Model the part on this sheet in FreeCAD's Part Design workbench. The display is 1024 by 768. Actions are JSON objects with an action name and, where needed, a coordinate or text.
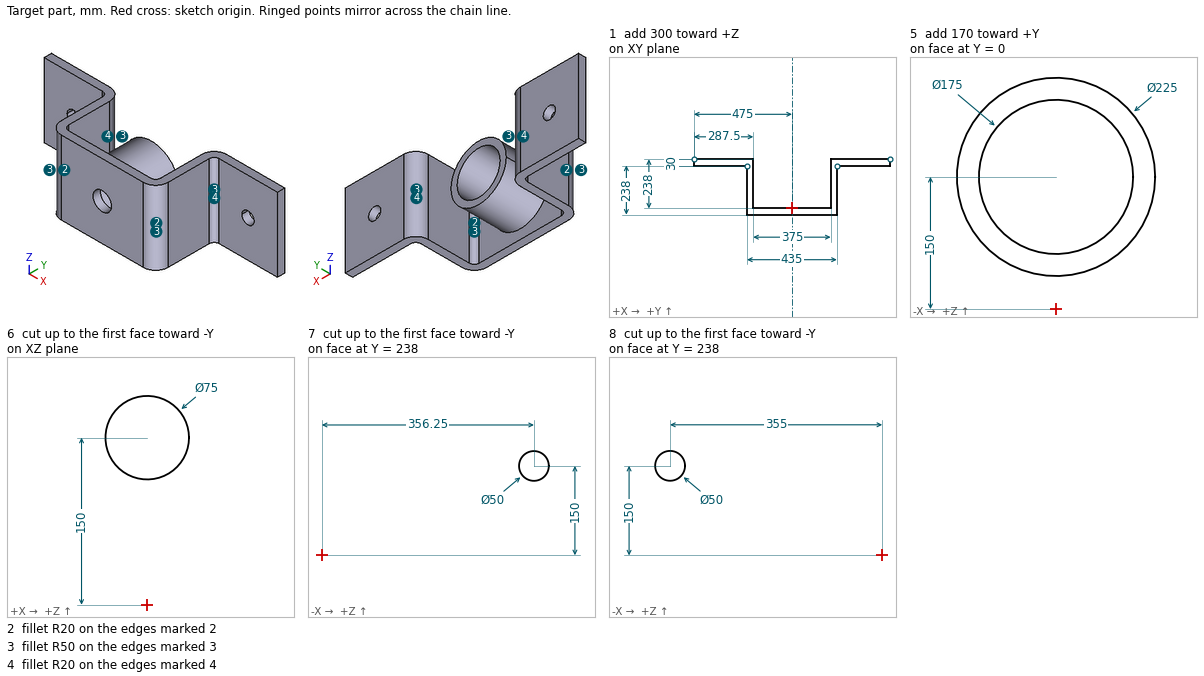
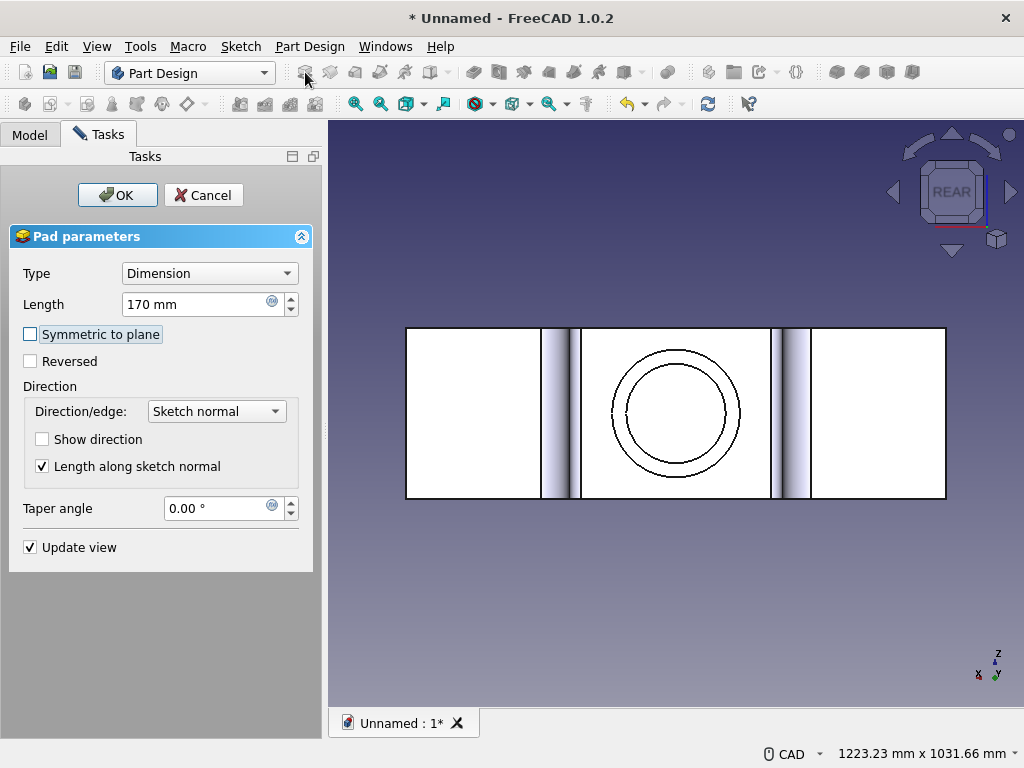
{"action": "left_click", "coordinate": [118, 195]}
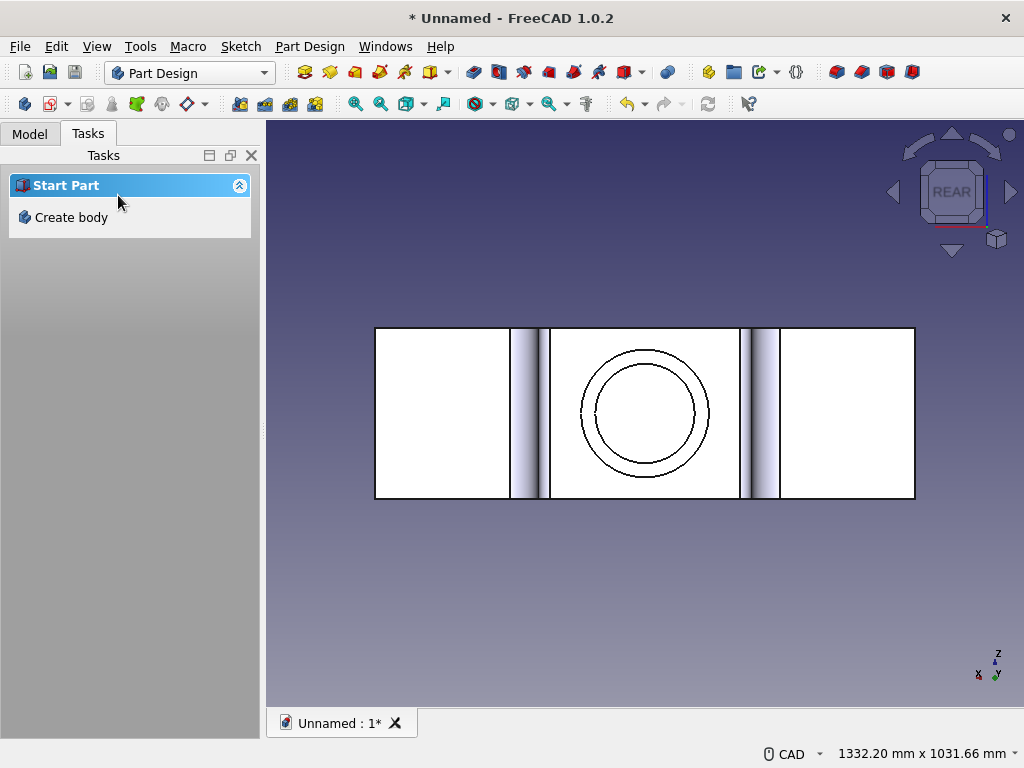
{"action": "left_click", "coordinate": [50, 104]}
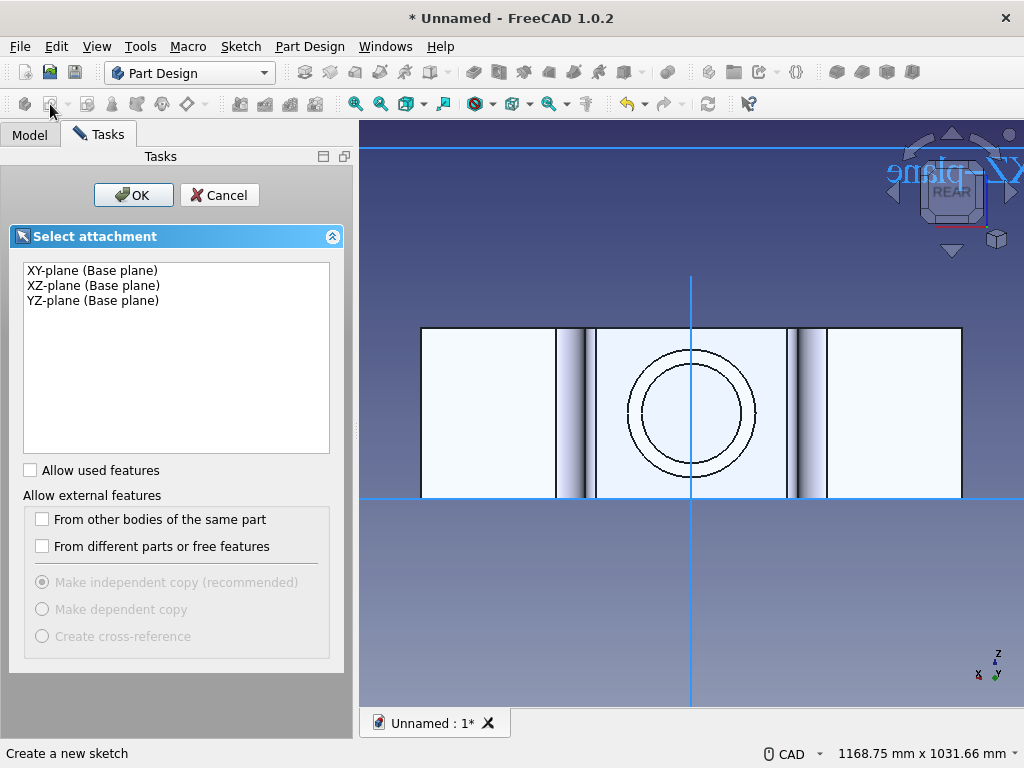
{"action": "left_click", "coordinate": [84, 286]}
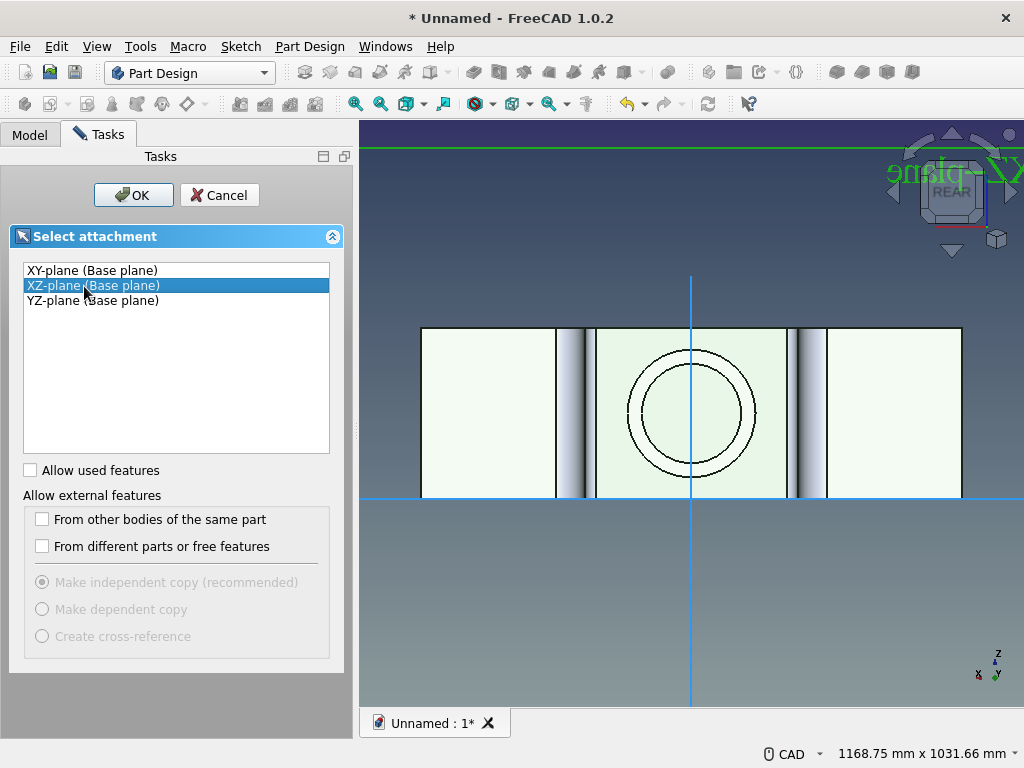
{"action": "left_click", "coordinate": [134, 195]}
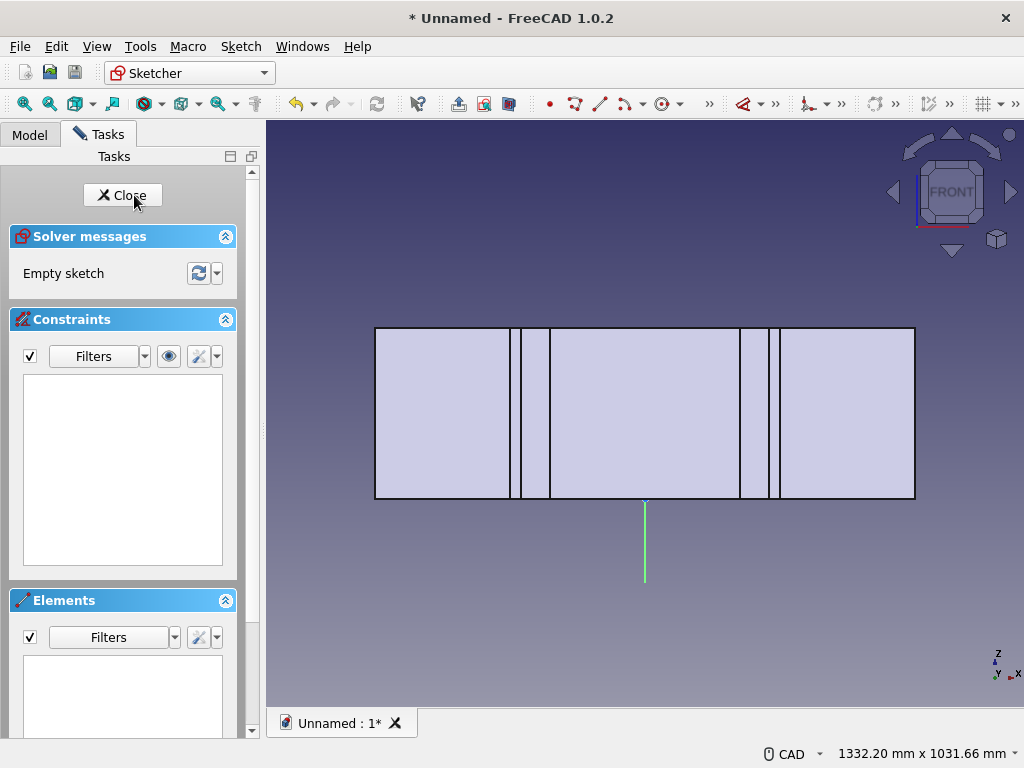
{"action": "left_click", "coordinate": [509, 104]}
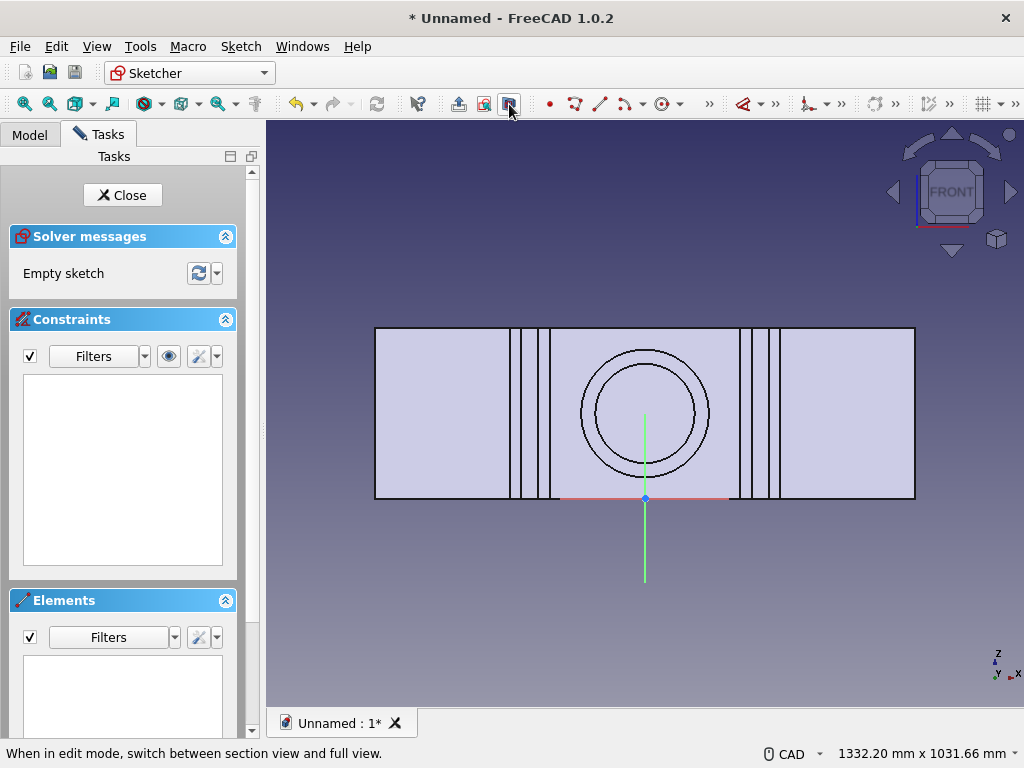
{"action": "scroll", "coordinate": [654, 414], "scroll_direction": "up", "scroll_amount": 11}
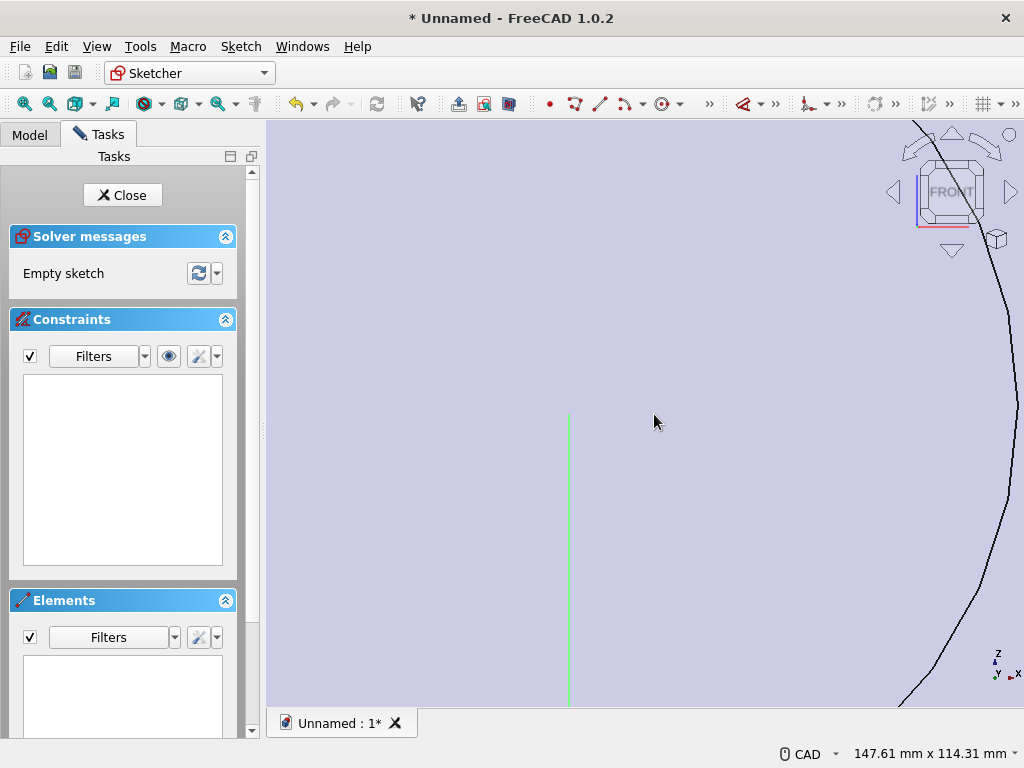
{"action": "left_click", "coordinate": [662, 104]}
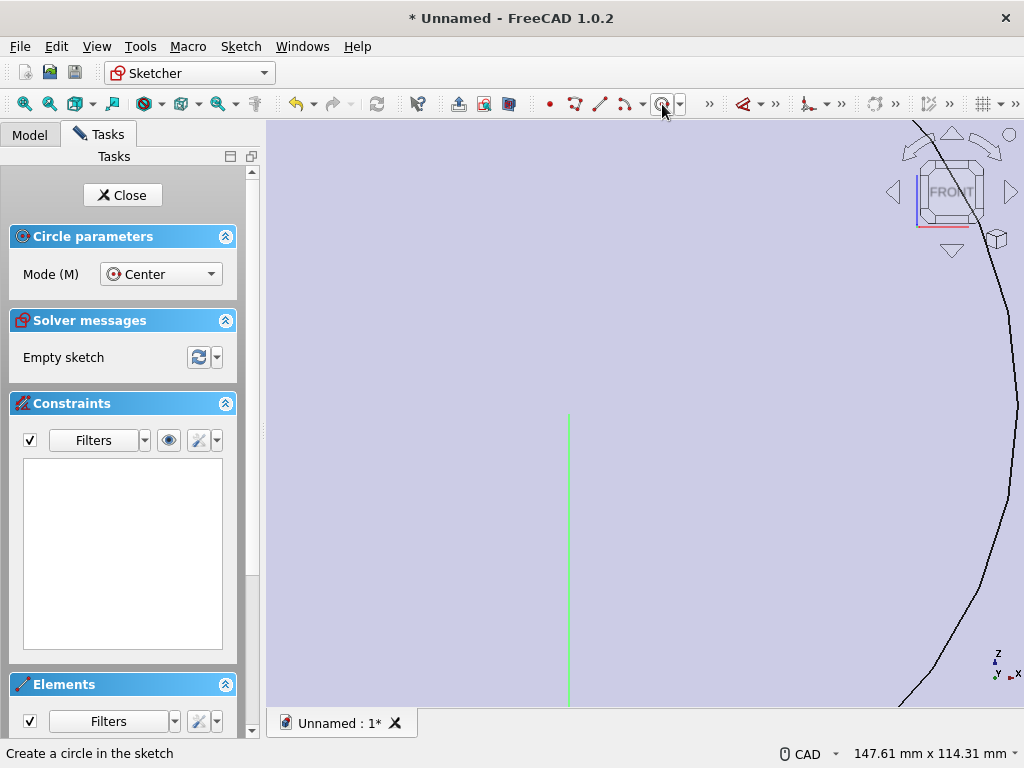
{"action": "left_click", "coordinate": [569, 405]}
{"action": "left_click", "coordinate": [705, 269]}
{"action": "key", "text": "Escape"}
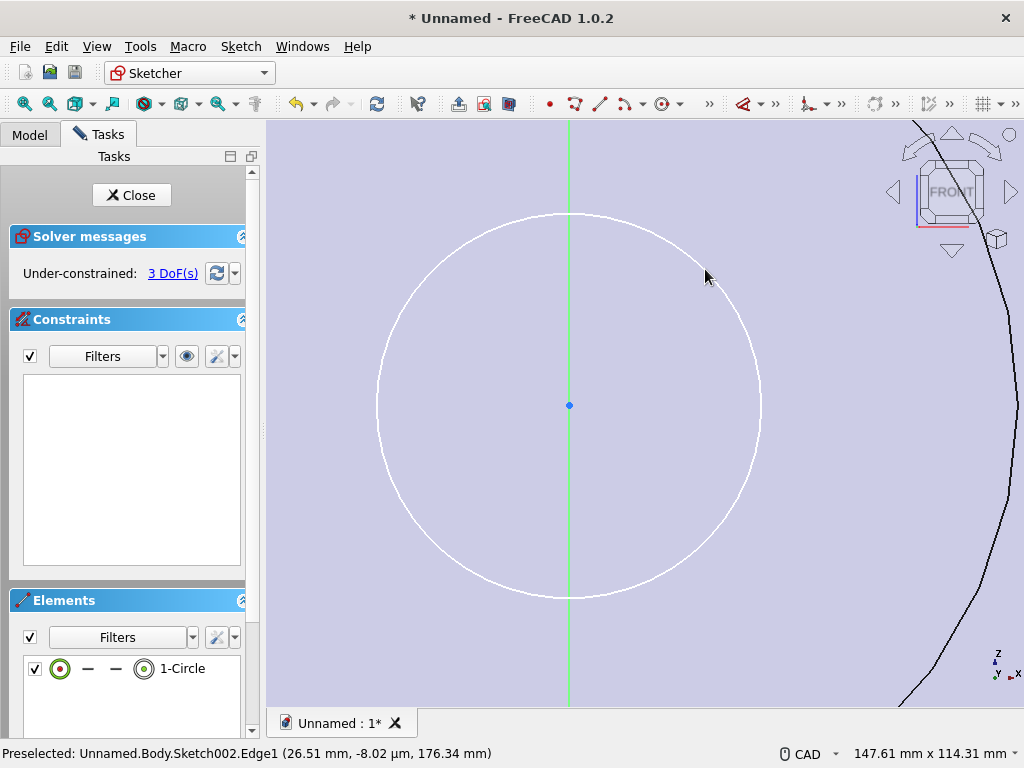
{"action": "left_click", "coordinate": [569, 406]}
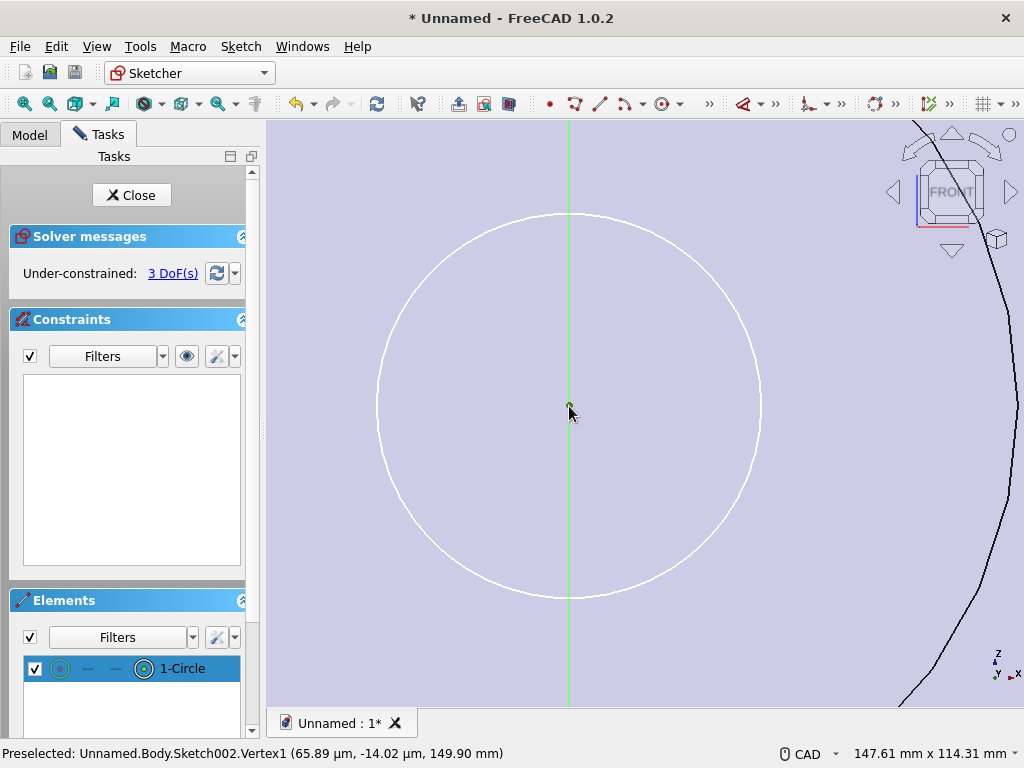
{"action": "left_click", "coordinate": [569, 641]}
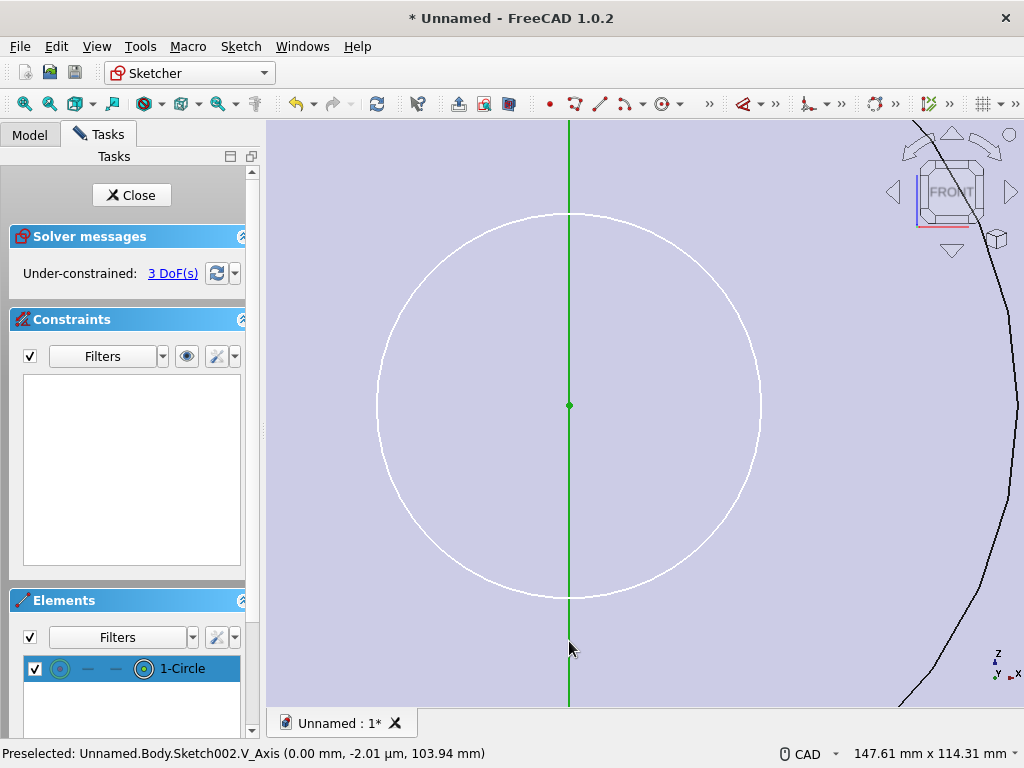
{"action": "key", "text": "c"}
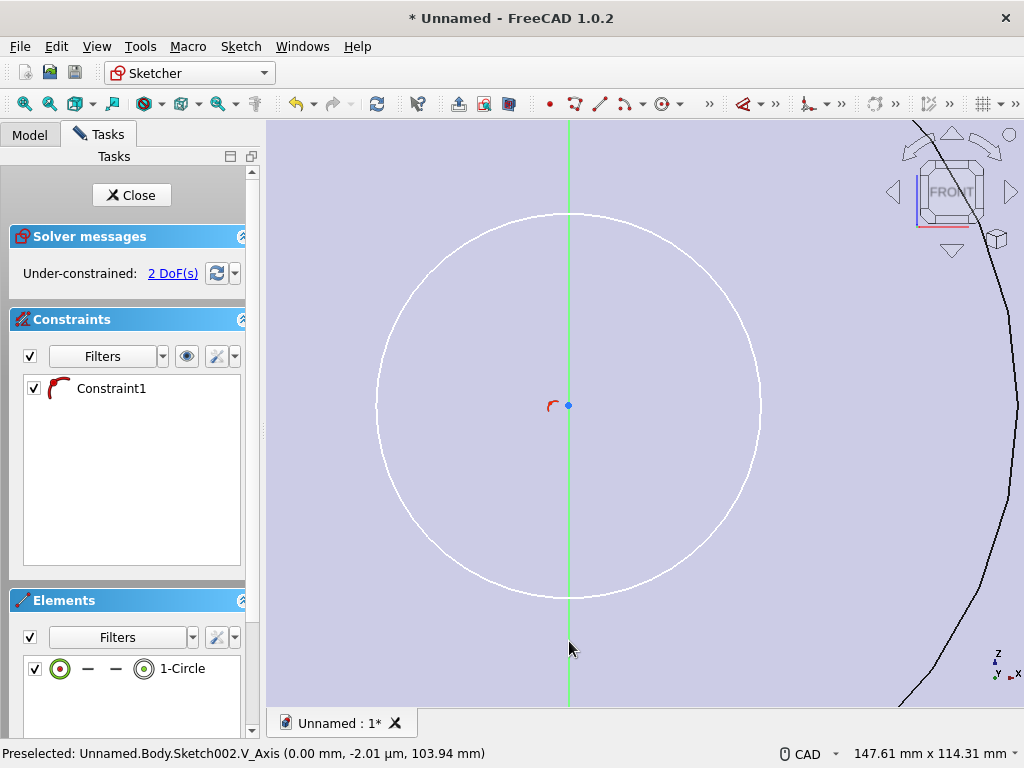
{"action": "key", "text": "d"}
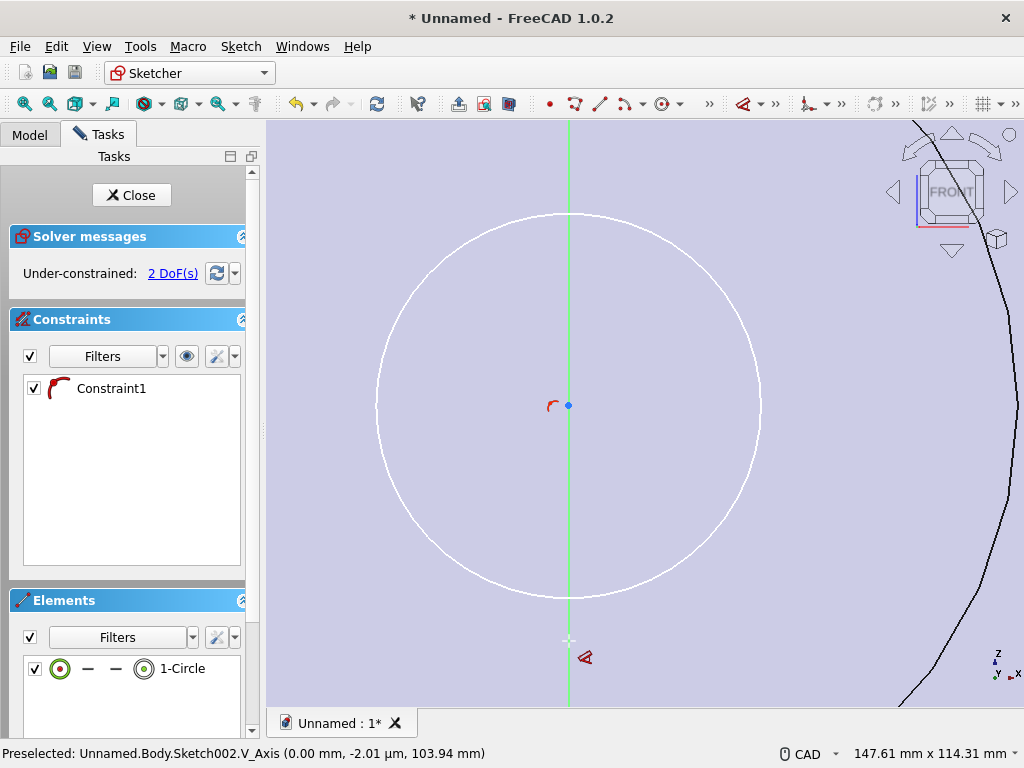
{"action": "left_click", "coordinate": [704, 270]}
{"action": "left_click", "coordinate": [727, 247]}